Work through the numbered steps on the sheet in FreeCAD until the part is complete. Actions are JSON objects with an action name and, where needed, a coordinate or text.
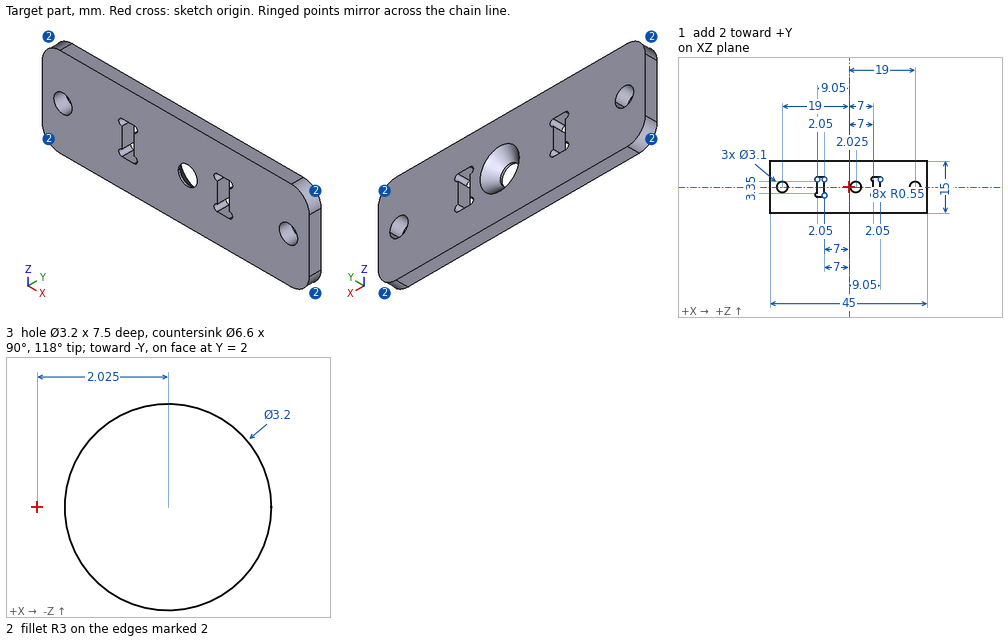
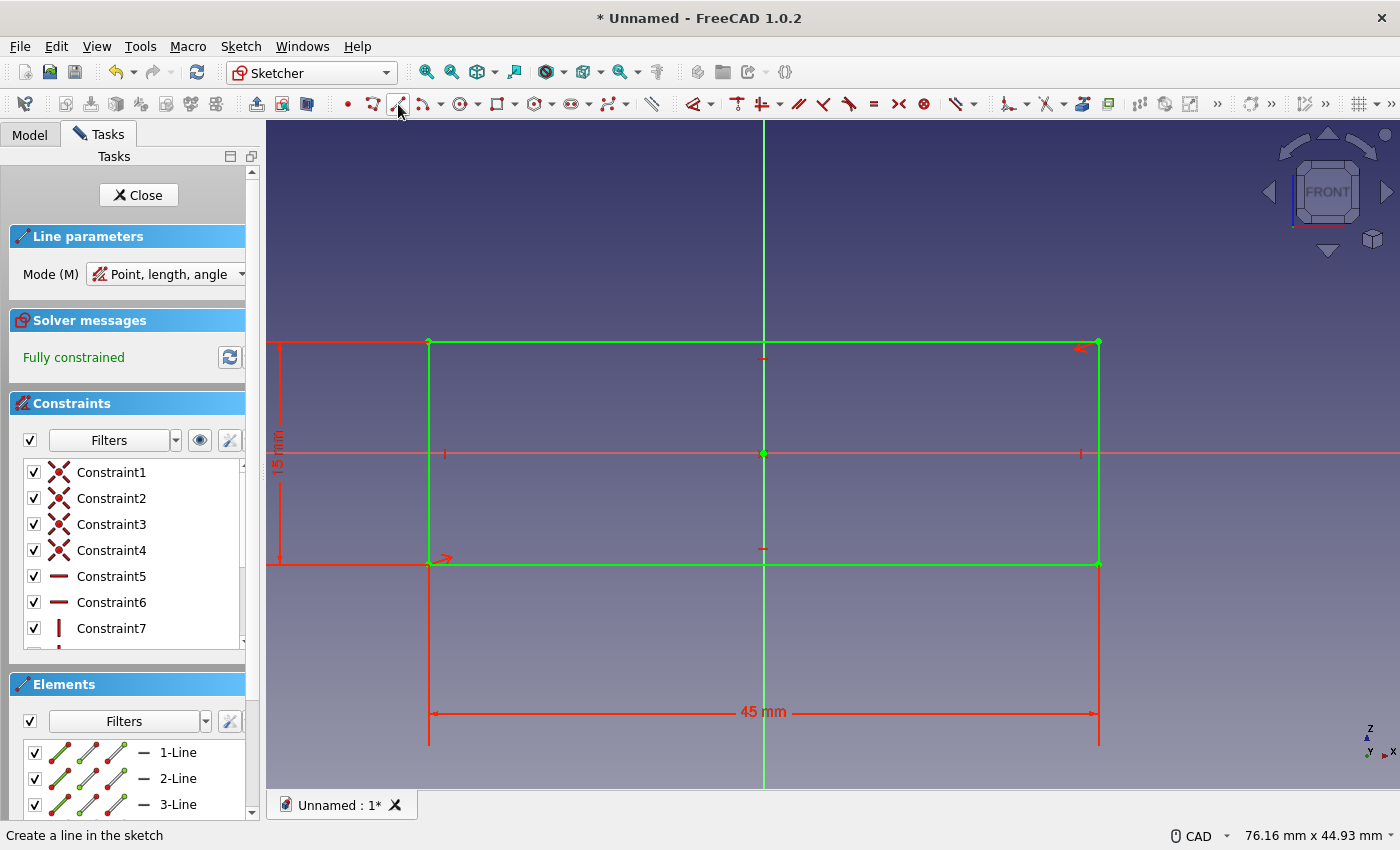
{"action": "left_click", "coordinate": [629, 428]}
{"action": "left_click", "coordinate": [629, 478]}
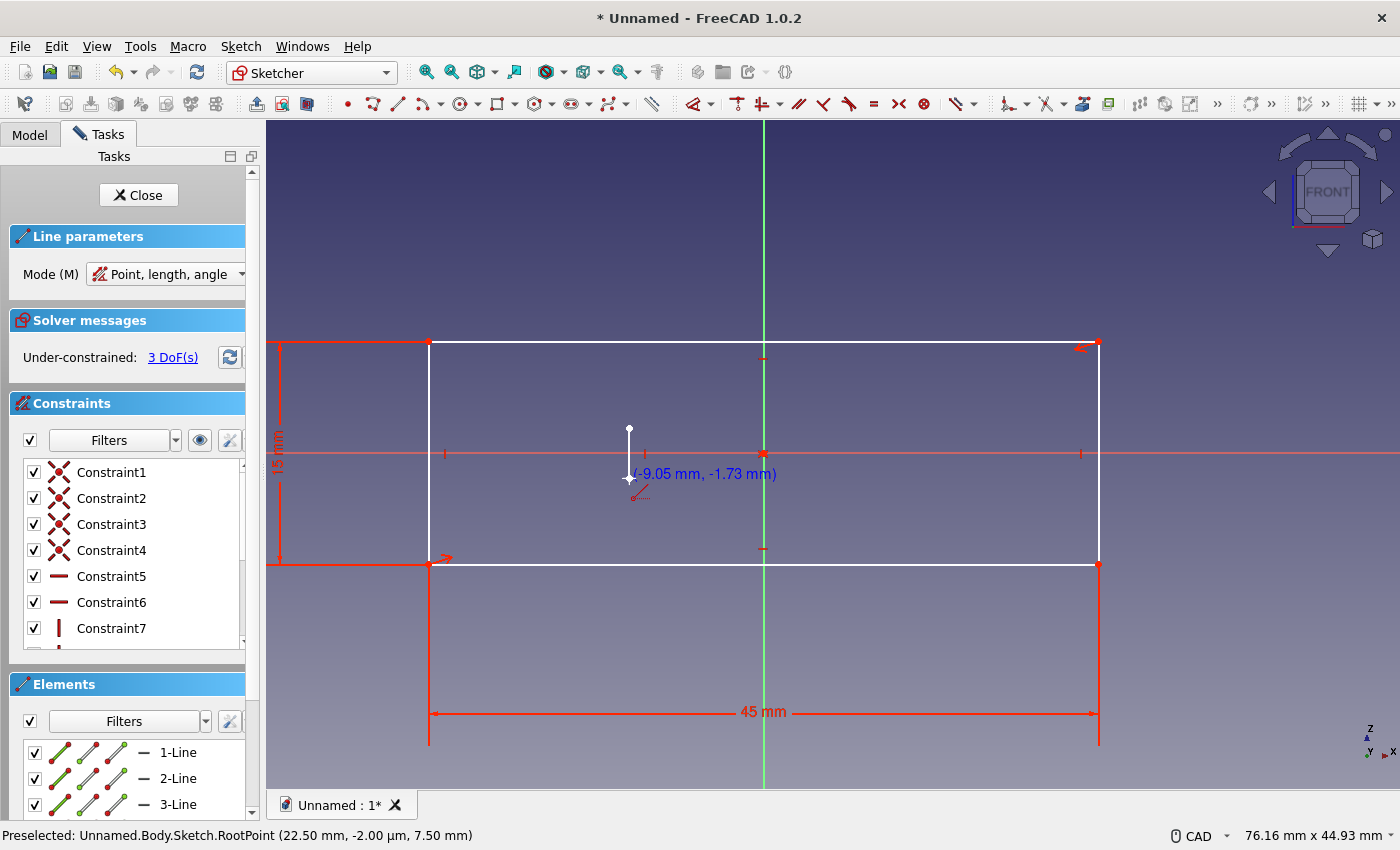
{"action": "left_click", "coordinate": [629, 495]}
{"action": "left_click", "coordinate": [659, 495]}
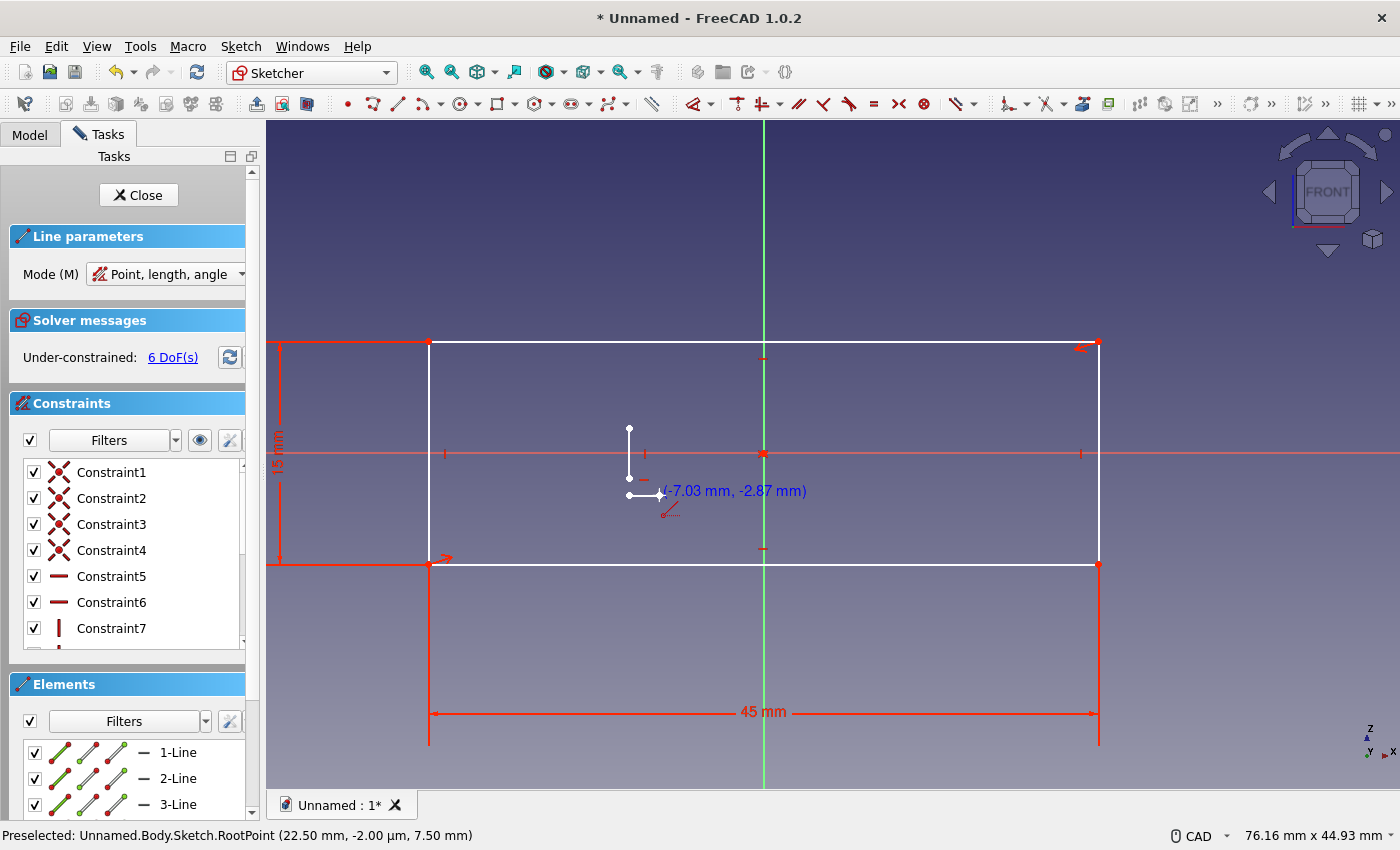
{"action": "left_click", "coordinate": [659, 478]}
{"action": "left_click", "coordinate": [659, 428]}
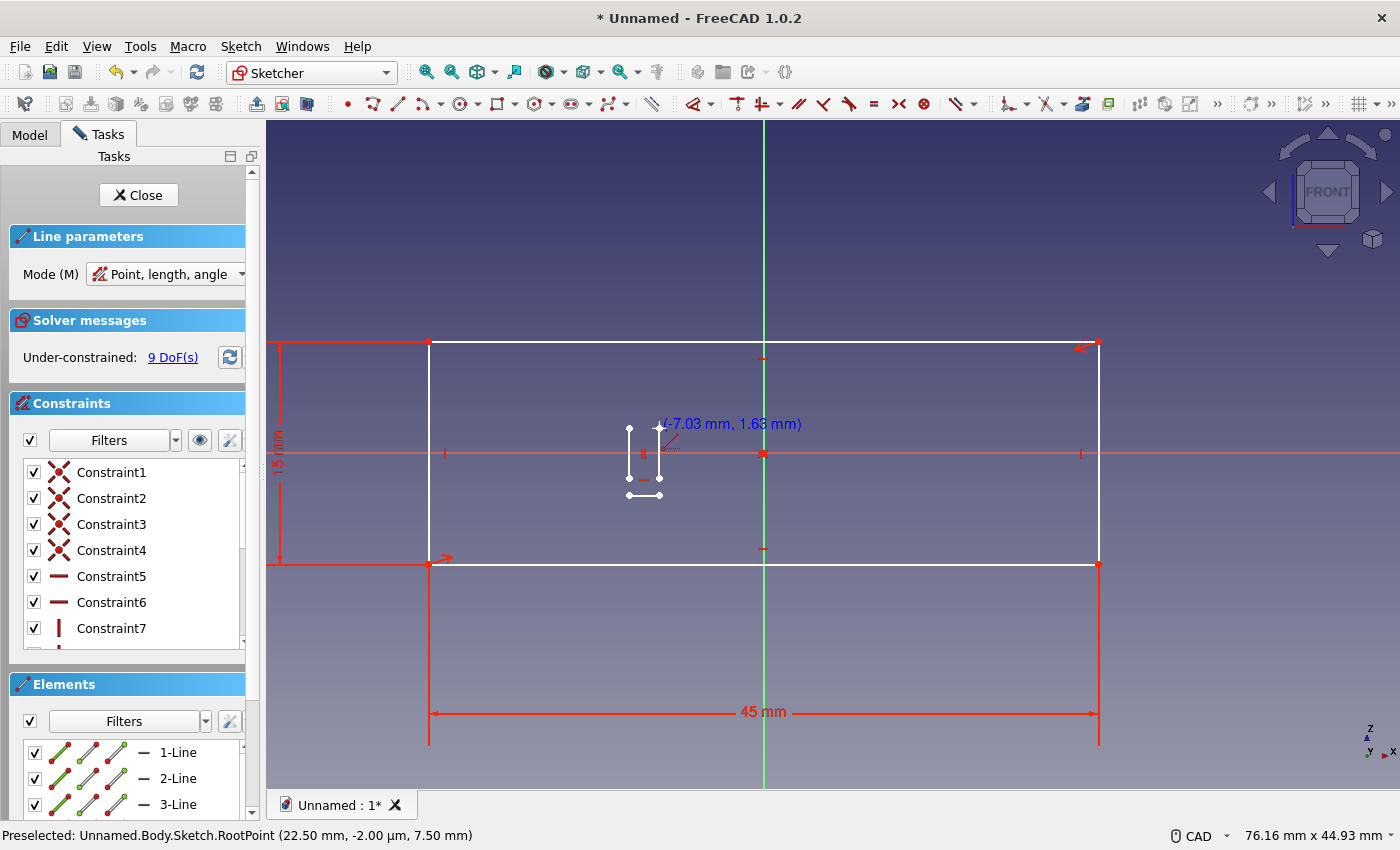
{"action": "left_click", "coordinate": [659, 412]}
{"action": "left_click", "coordinate": [629, 412]}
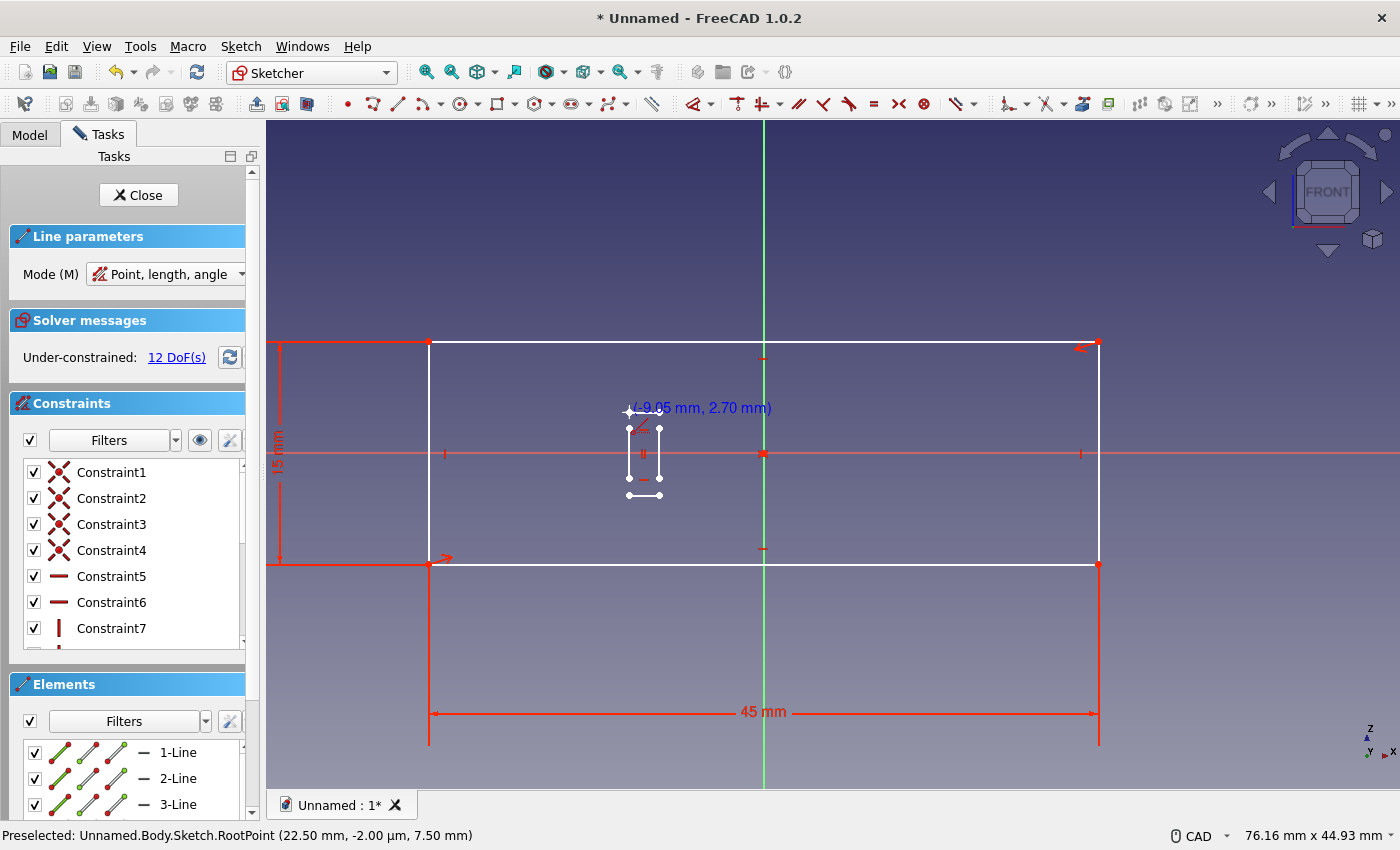
{"action": "key", "text": "g 3 a"}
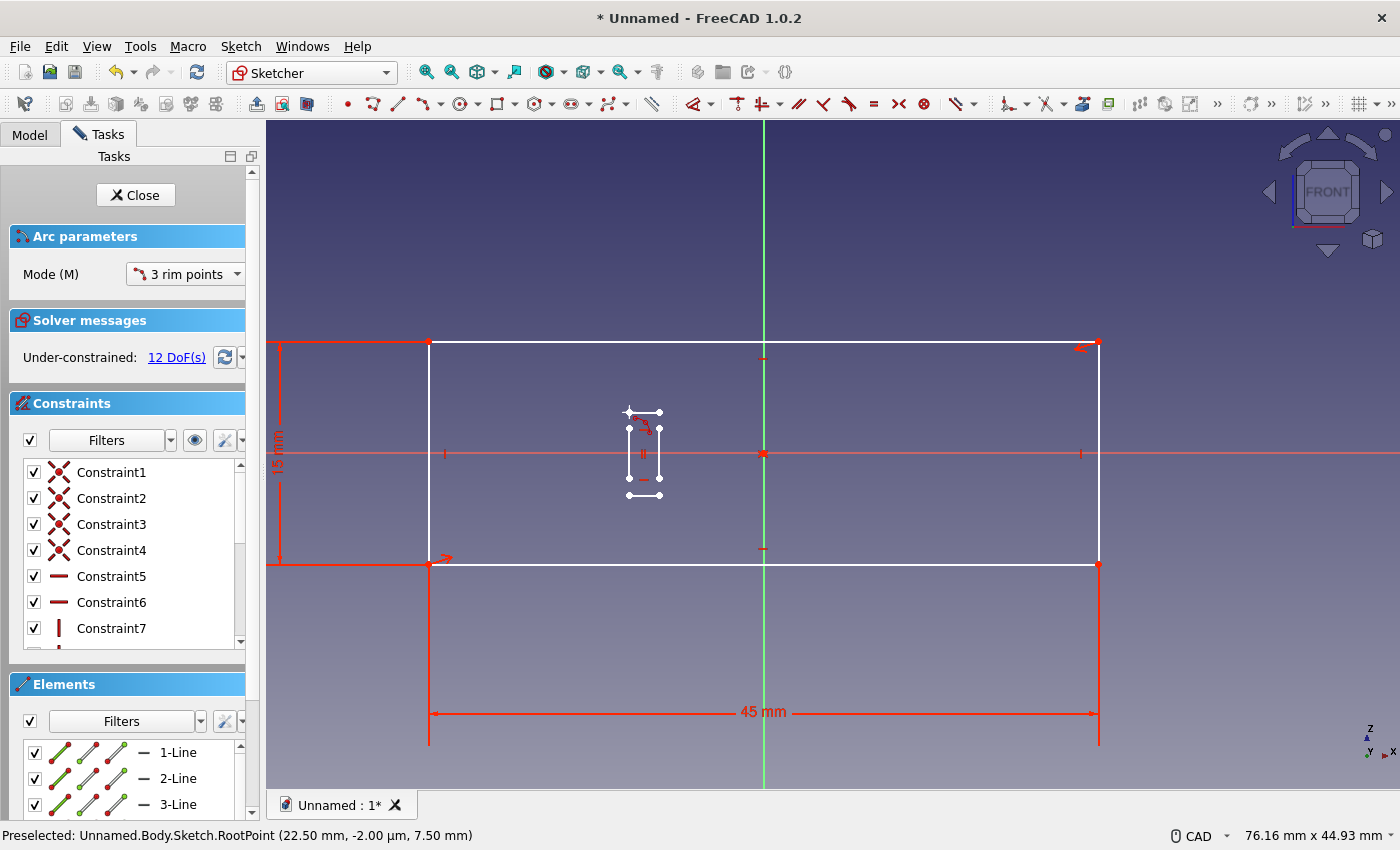
{"action": "left_click", "coordinate": [629, 479]}
{"action": "left_click", "coordinate": [629, 496]}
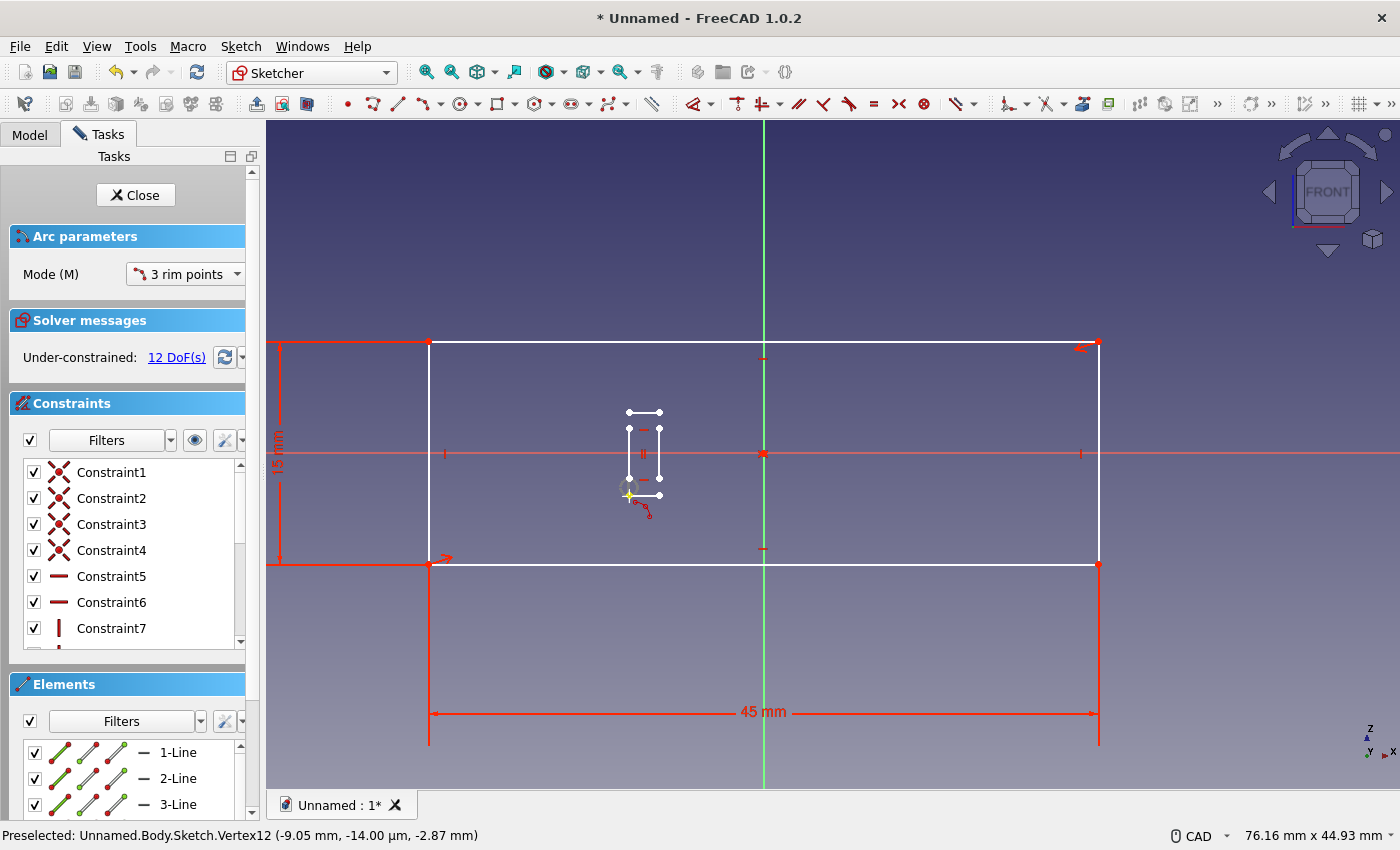
{"action": "scroll", "coordinate": [621, 486], "scroll_direction": "up", "scroll_amount": 4}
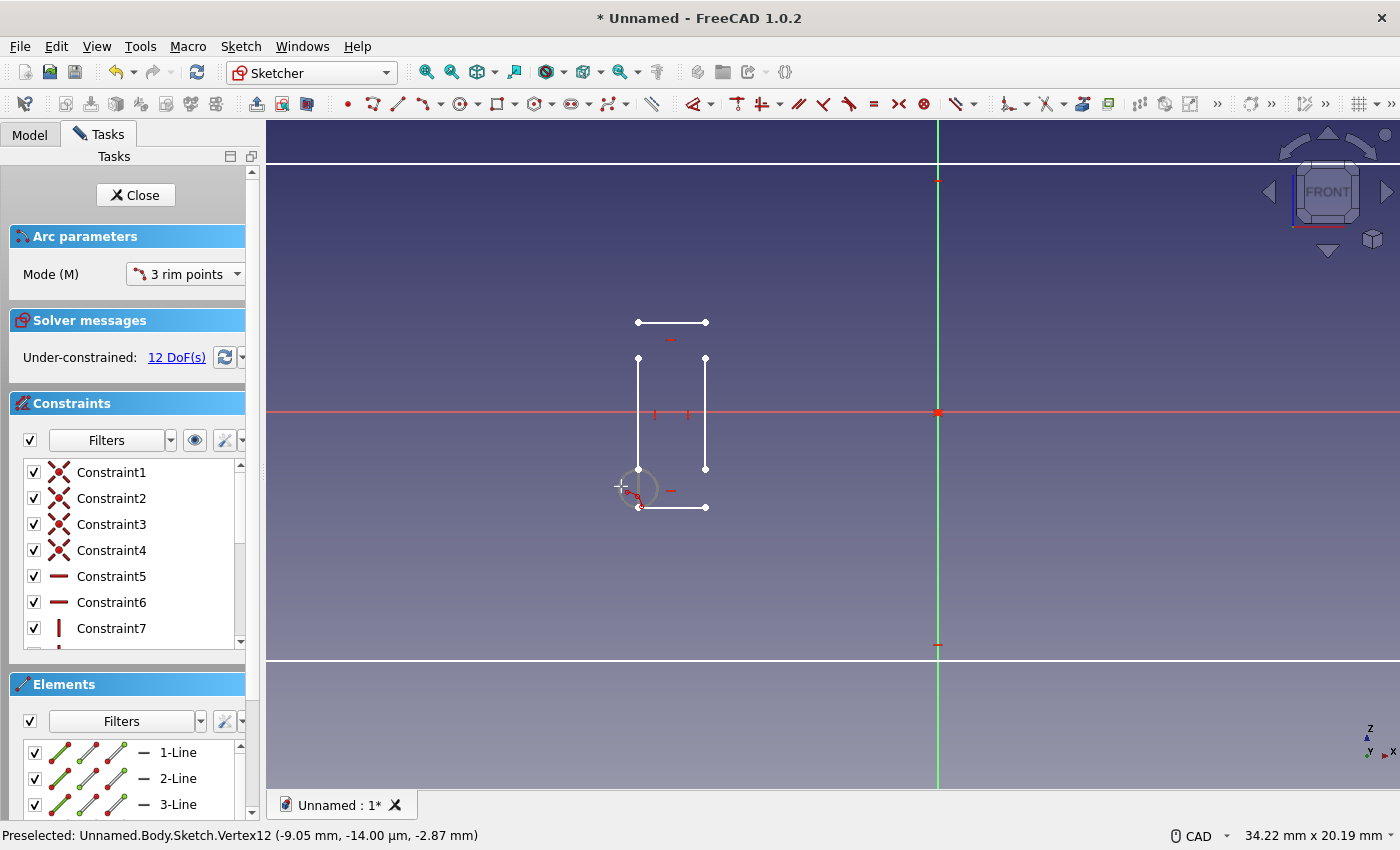
{"action": "left_click", "coordinate": [620, 486]}